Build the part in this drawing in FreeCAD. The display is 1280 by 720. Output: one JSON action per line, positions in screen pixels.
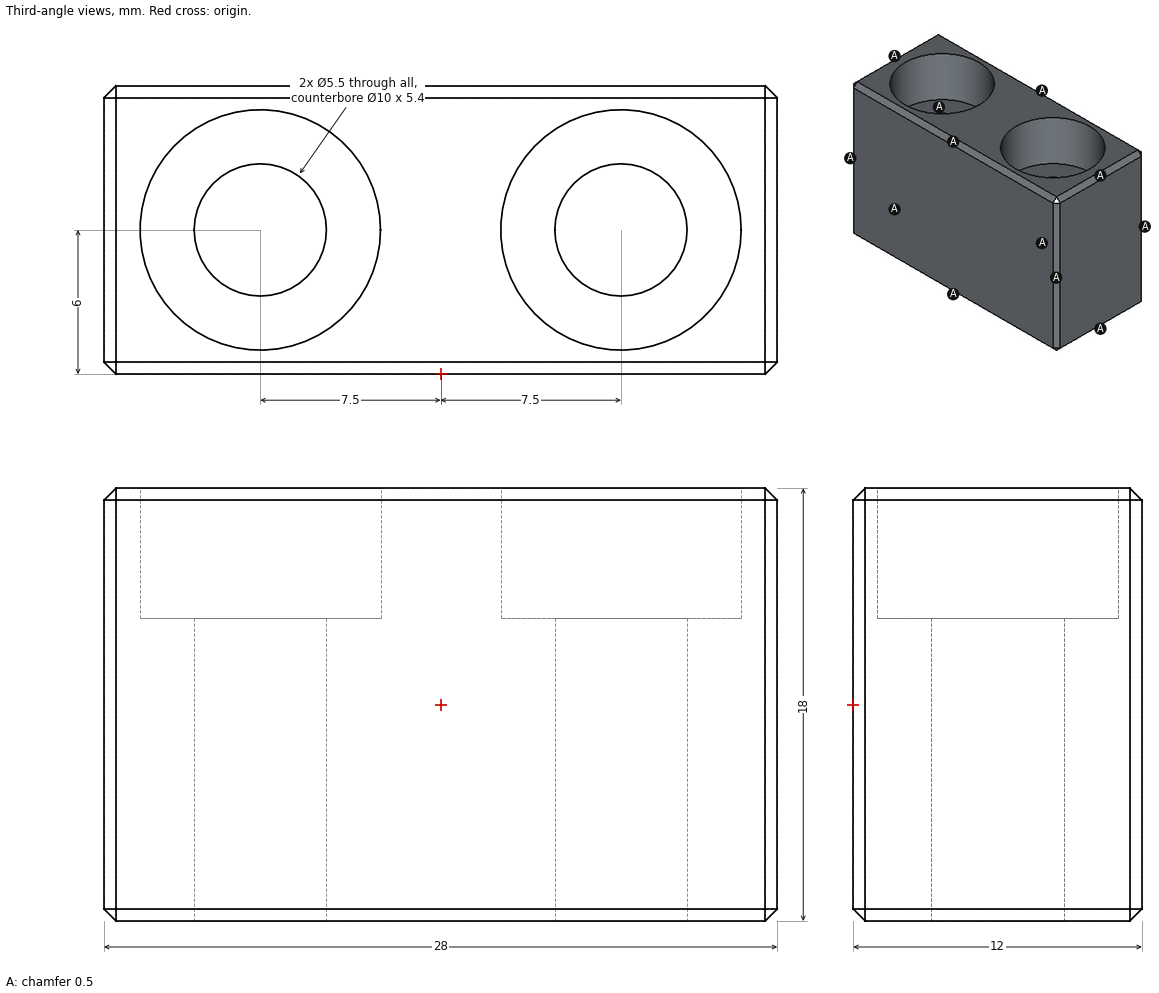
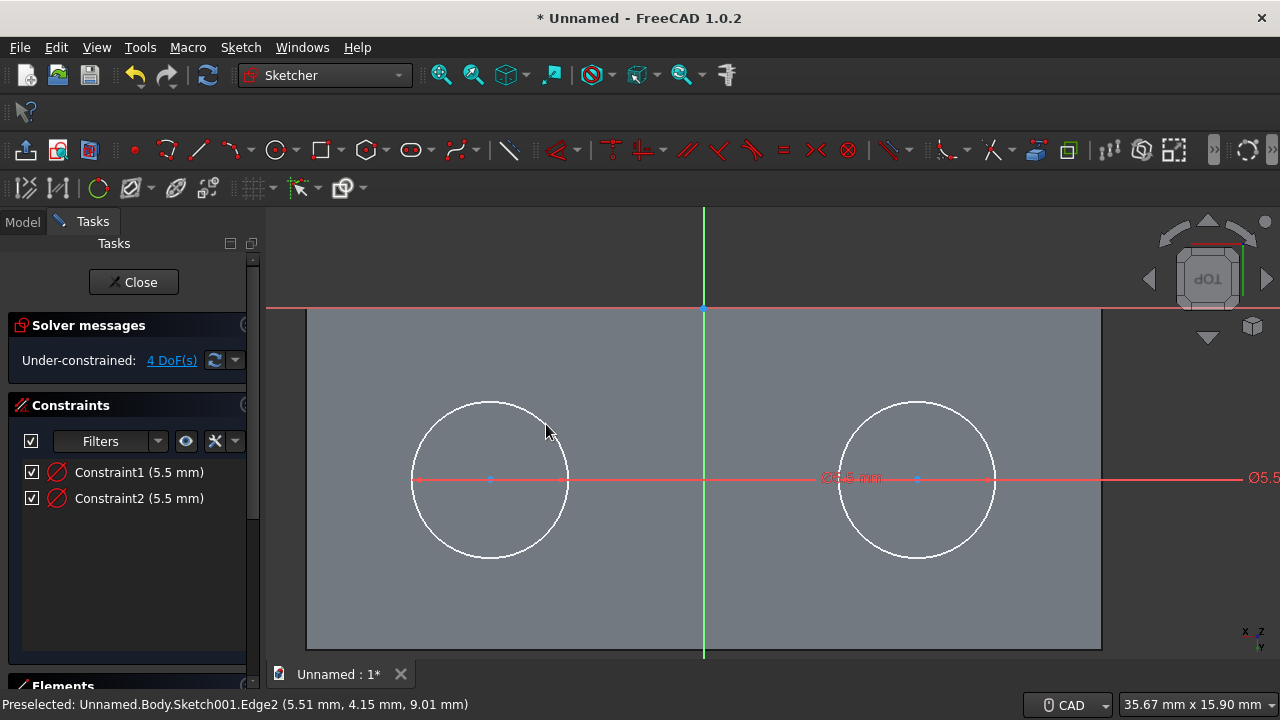
{"action": "left_click", "coordinate": [917, 480]}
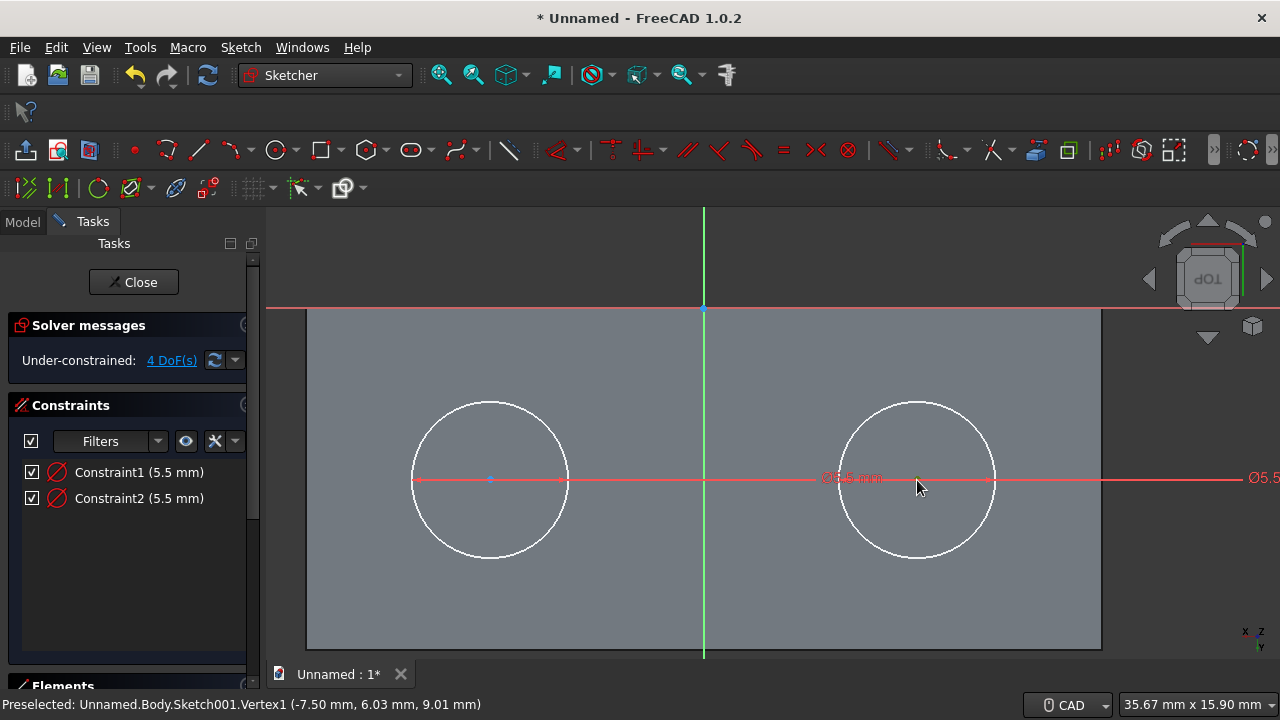
{"action": "left_click", "coordinate": [490, 480]}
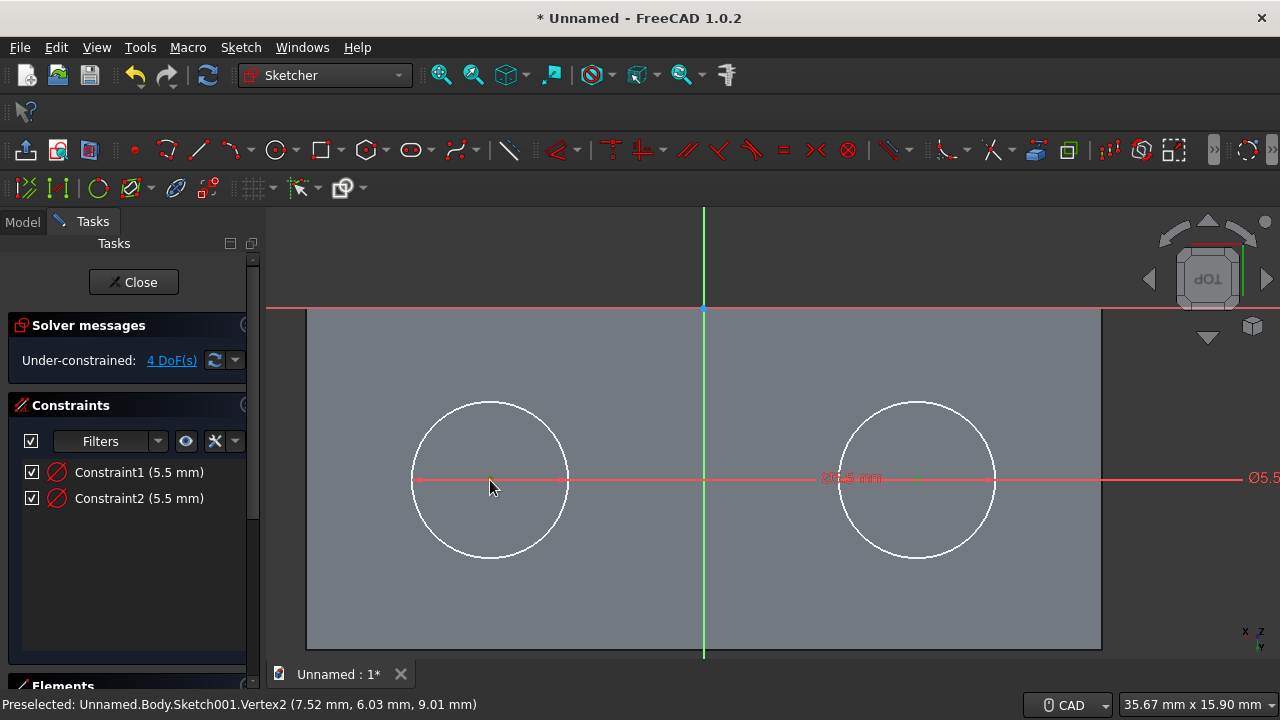
{"action": "key", "text": "h"}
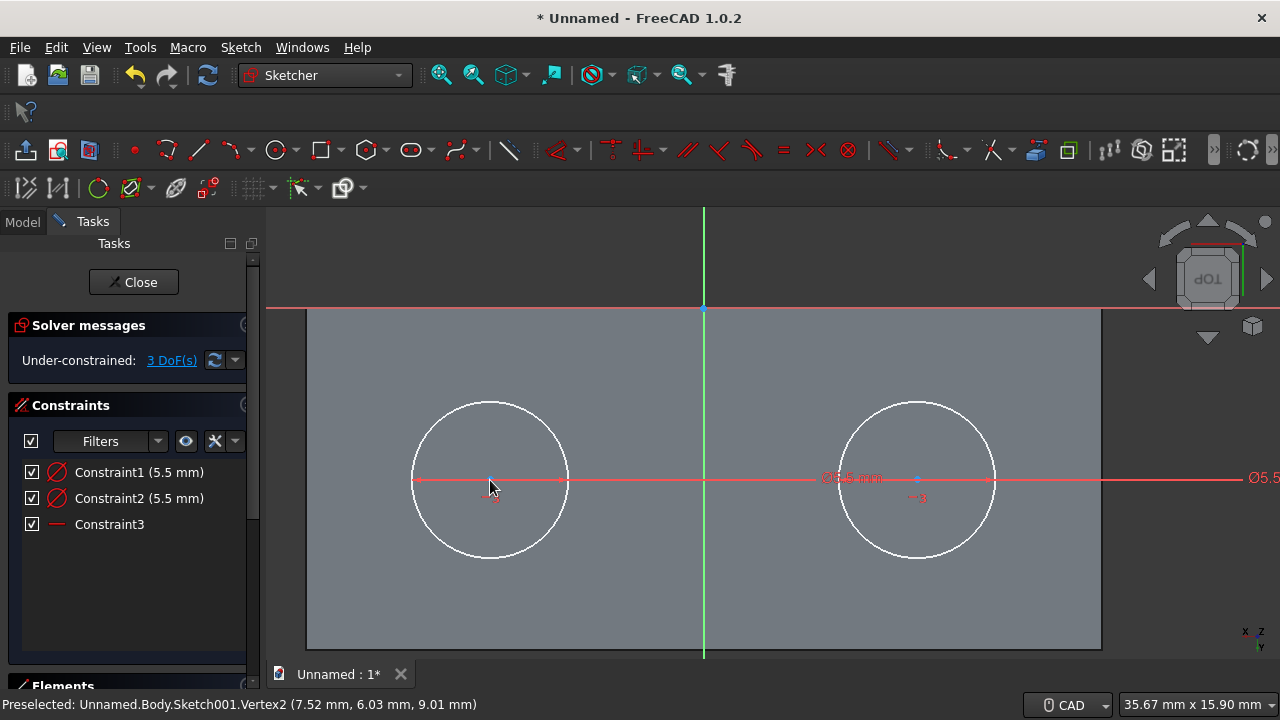
{"action": "left_click", "coordinate": [556, 150]}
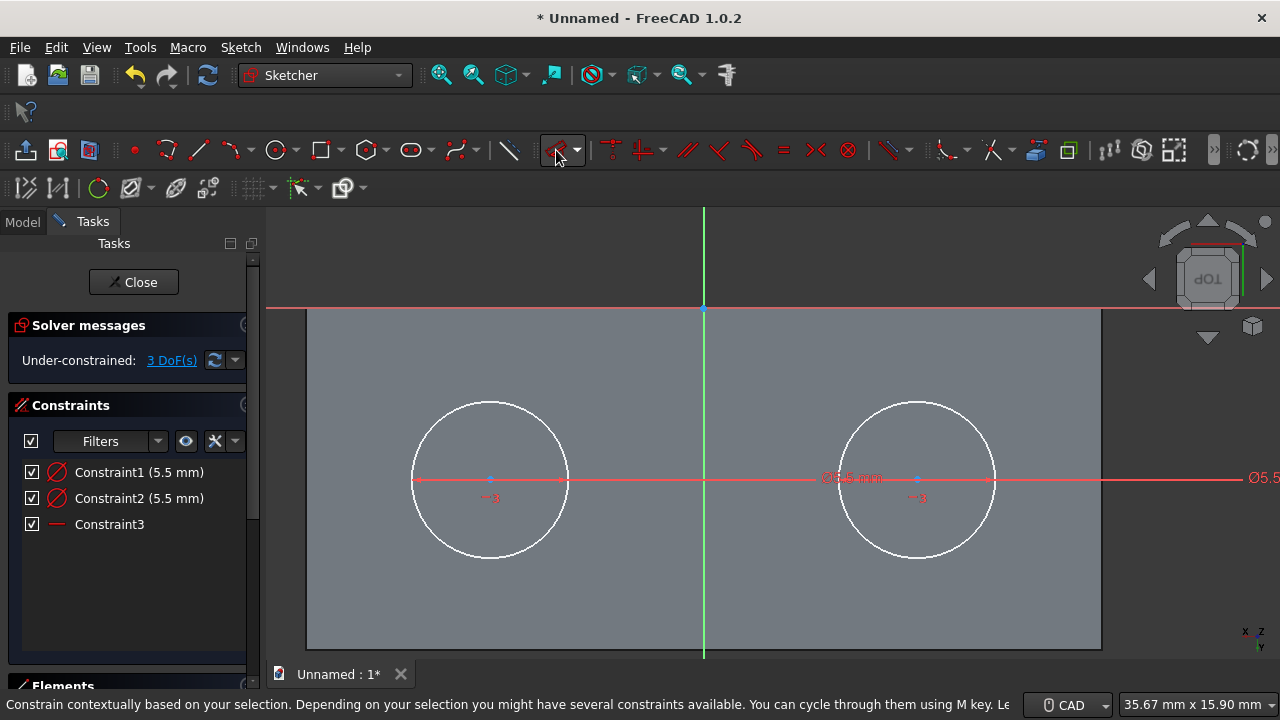
{"action": "left_click", "coordinate": [917, 480]}
{"action": "left_click", "coordinate": [951, 394]}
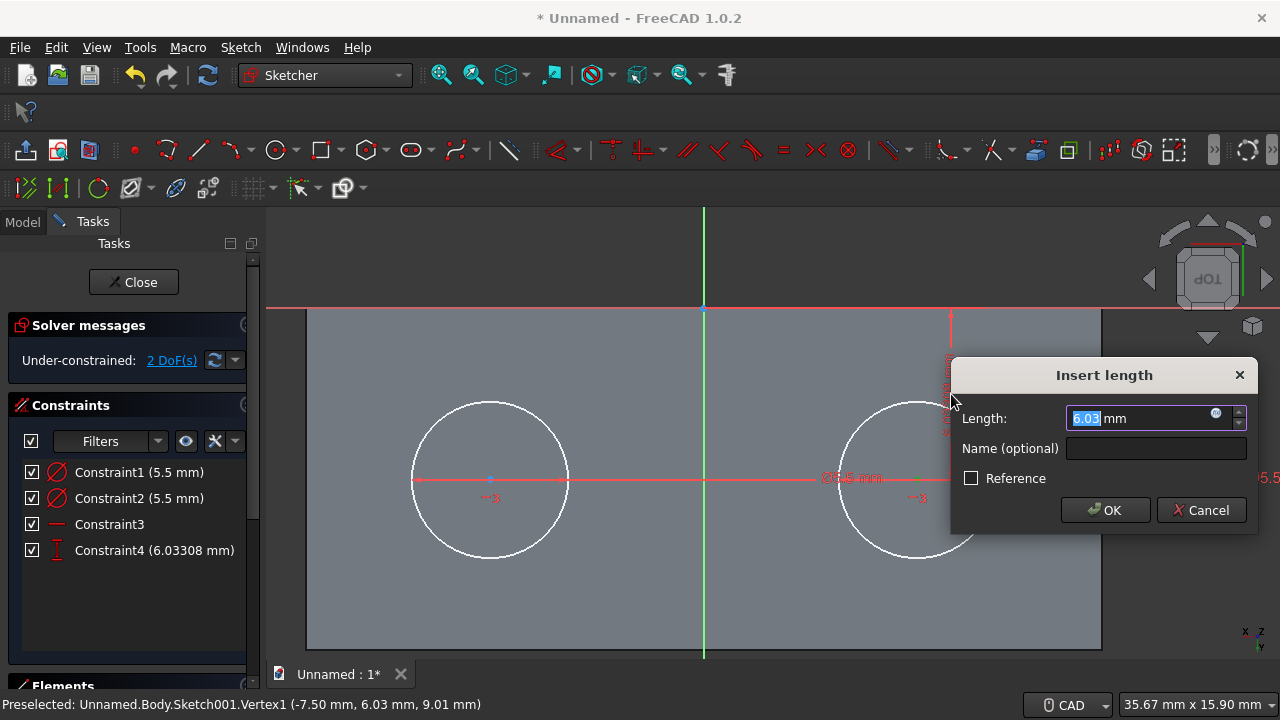
{"action": "type", "text": "6"}
{"action": "key", "text": "Return"}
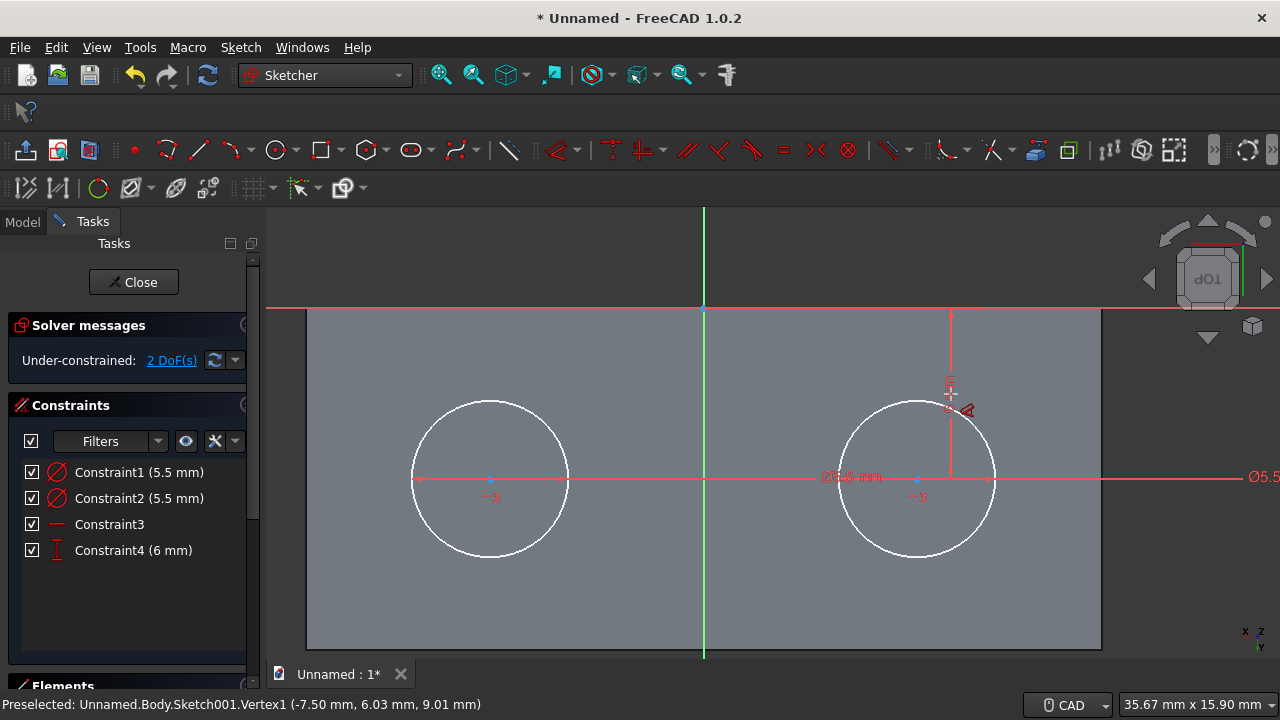
{"action": "left_click", "coordinate": [917, 479]}
{"action": "left_click", "coordinate": [810, 274]}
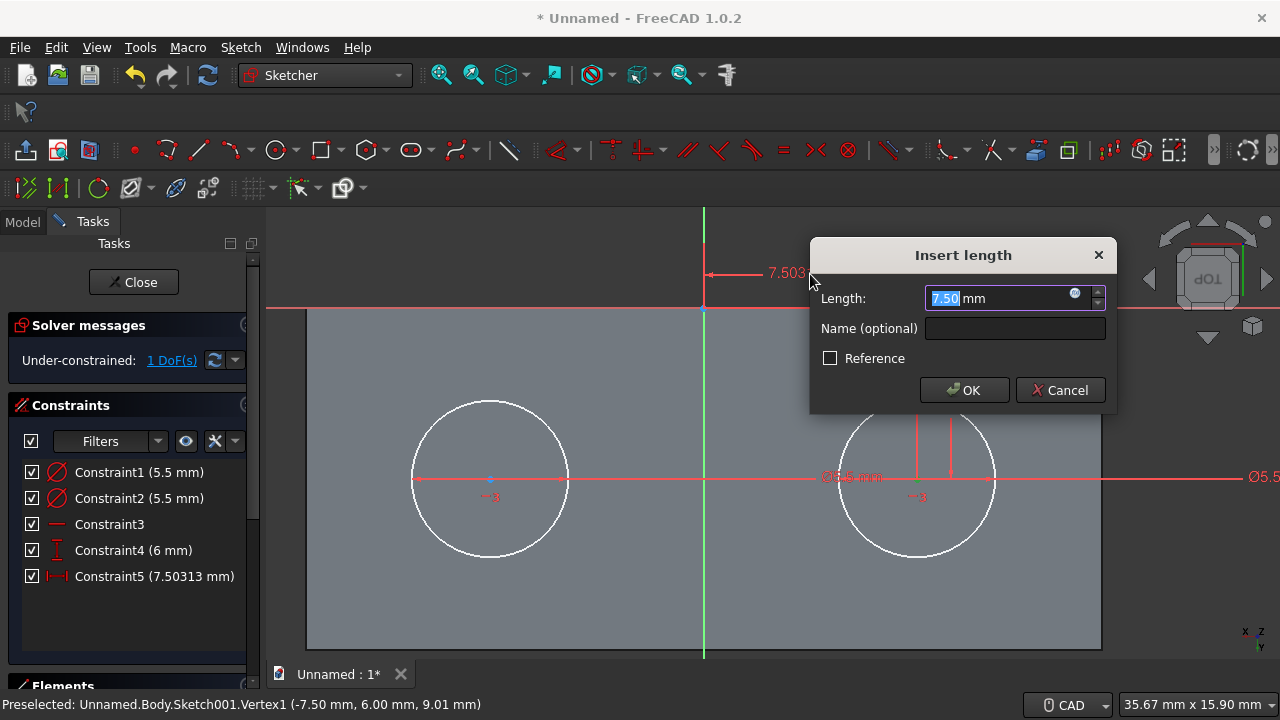
{"action": "type", "text": "7.5"}
{"action": "key", "text": "Return"}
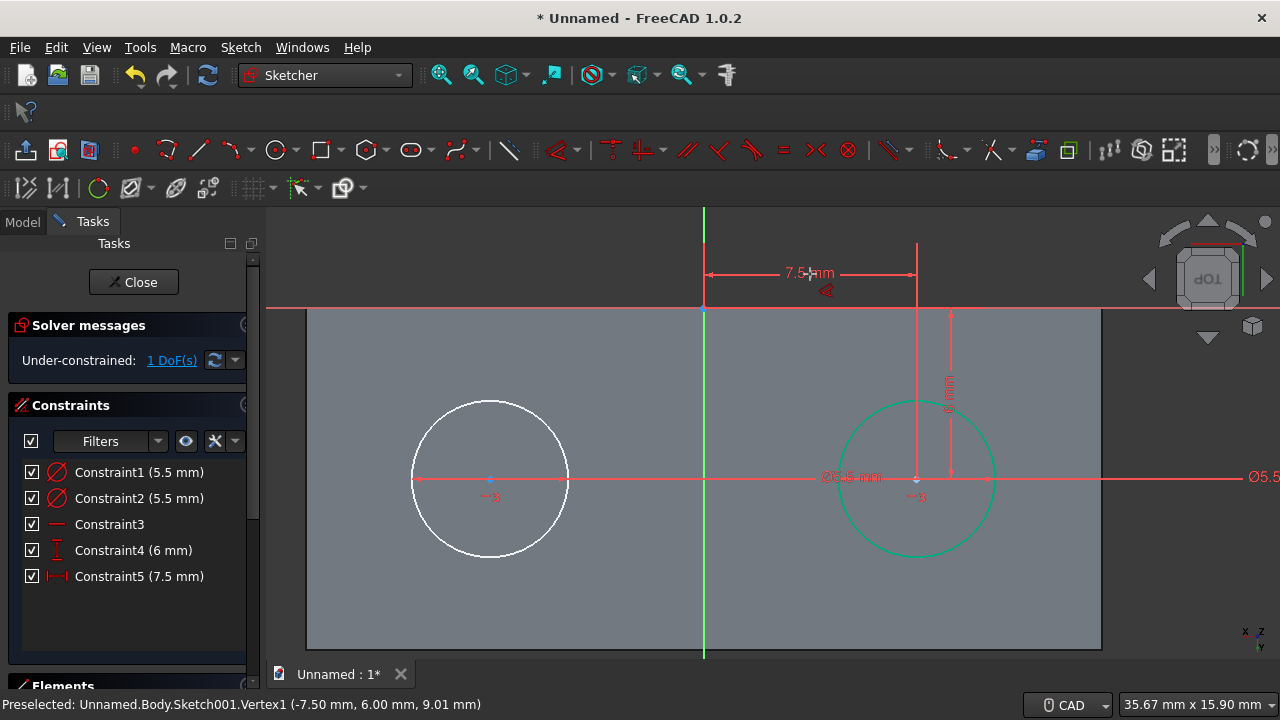
{"action": "left_click", "coordinate": [490, 479]}
{"action": "left_click", "coordinate": [597, 274]}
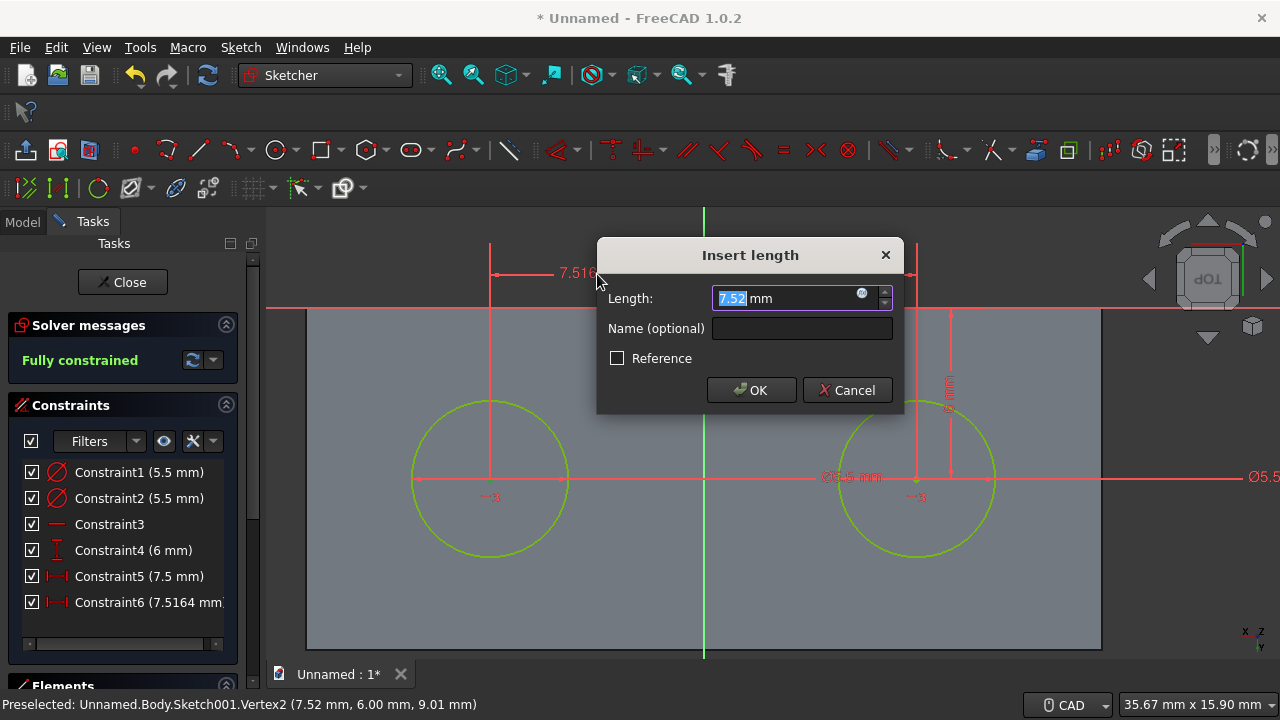
{"action": "type", "text": "7.5"}
{"action": "key", "text": "Return"}
{"action": "key", "text": "Escape"}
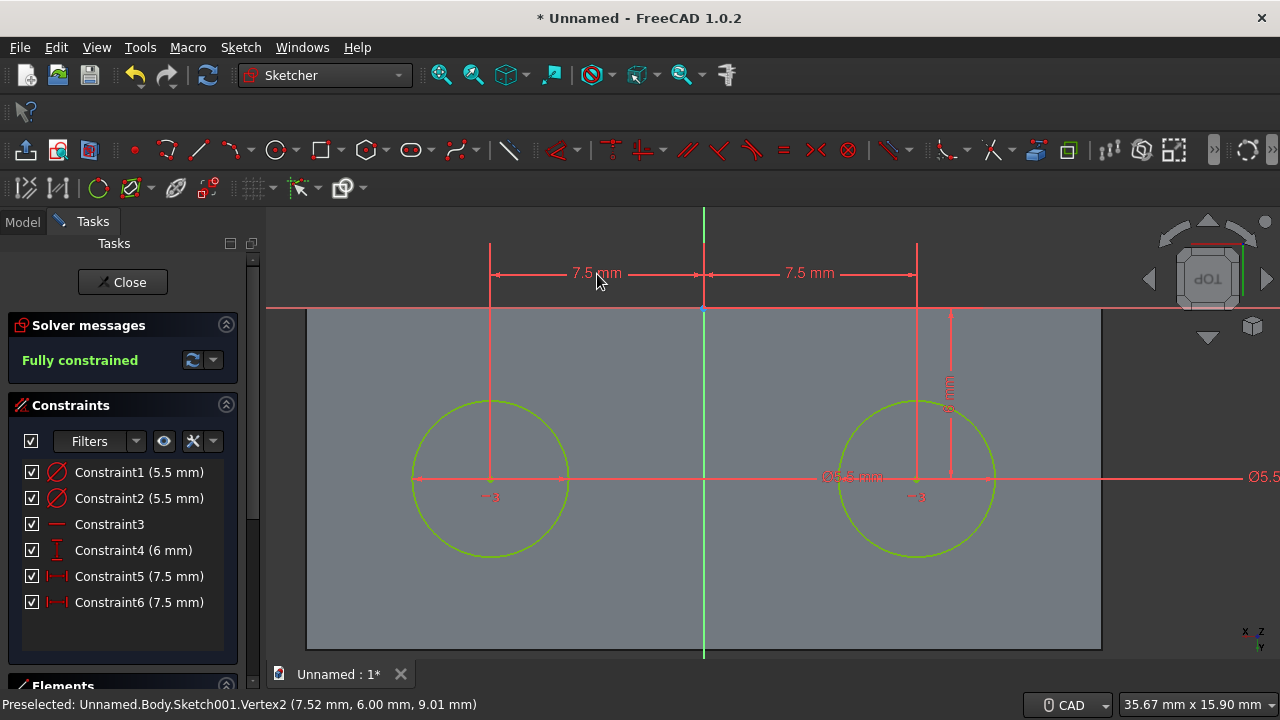
{"action": "left_click", "coordinate": [123, 282]}